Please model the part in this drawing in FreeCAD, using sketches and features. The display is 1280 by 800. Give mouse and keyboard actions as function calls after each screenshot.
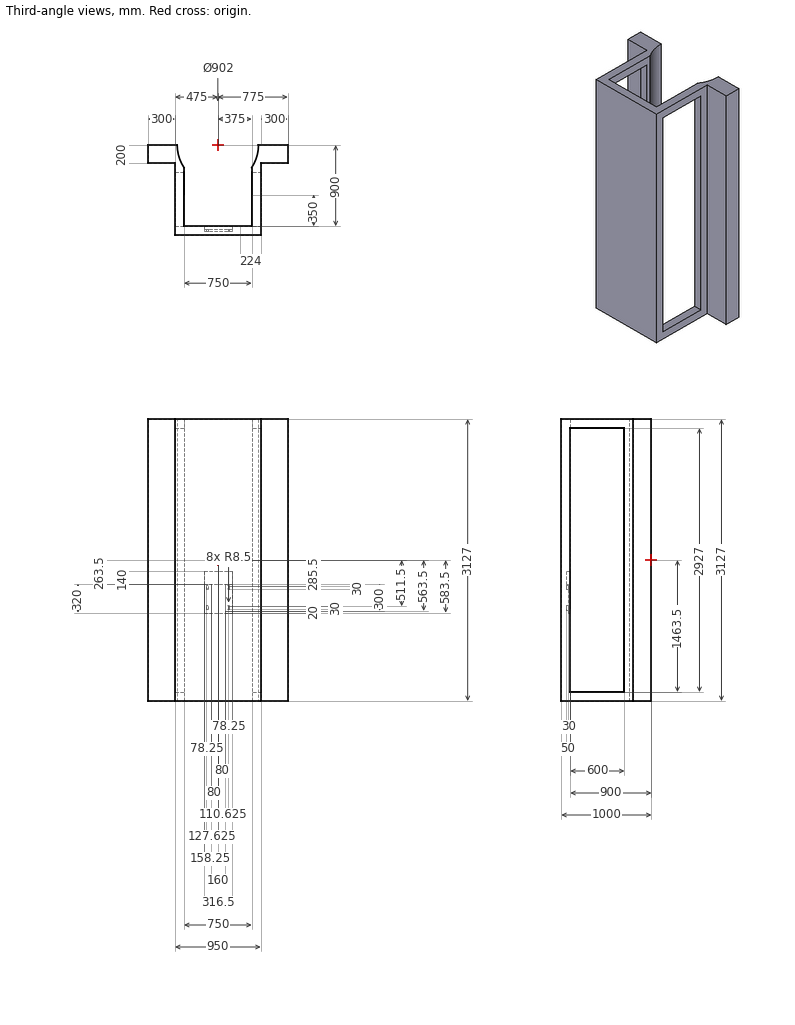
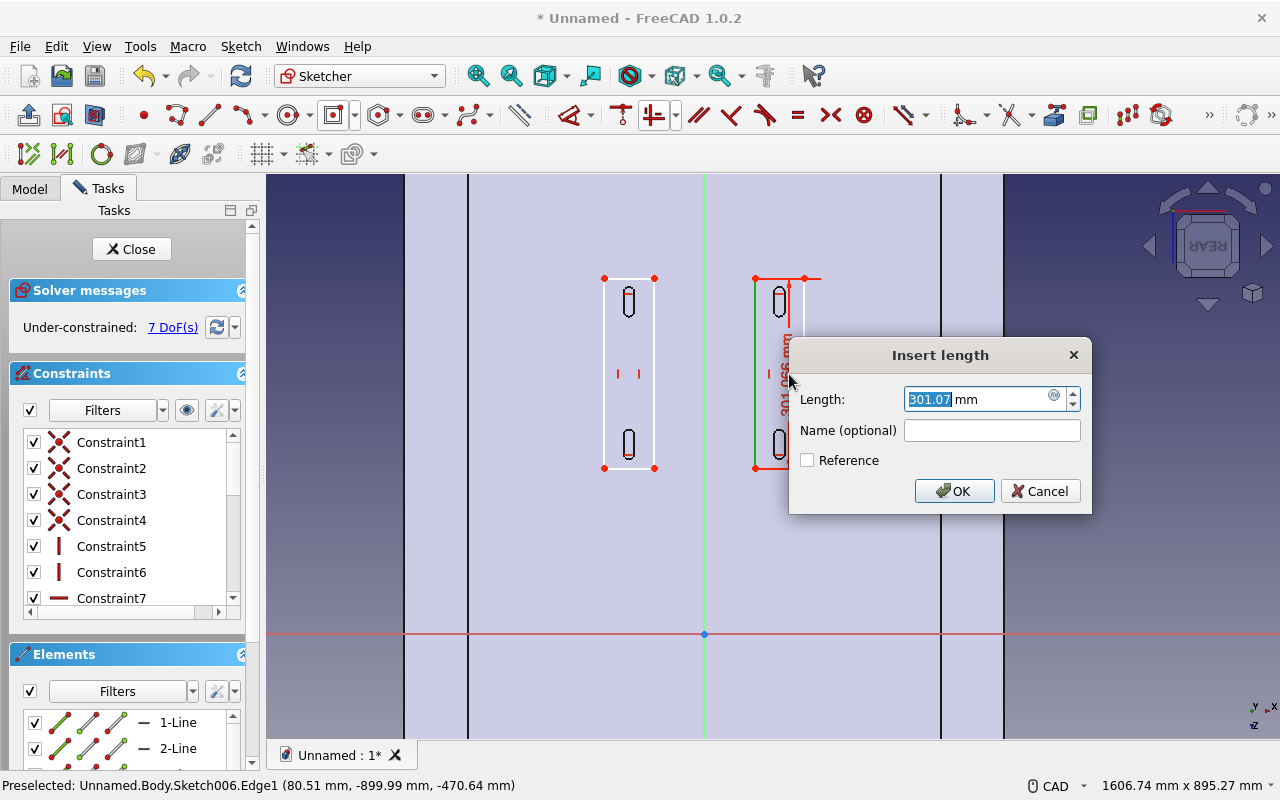
text(300)
key(Return)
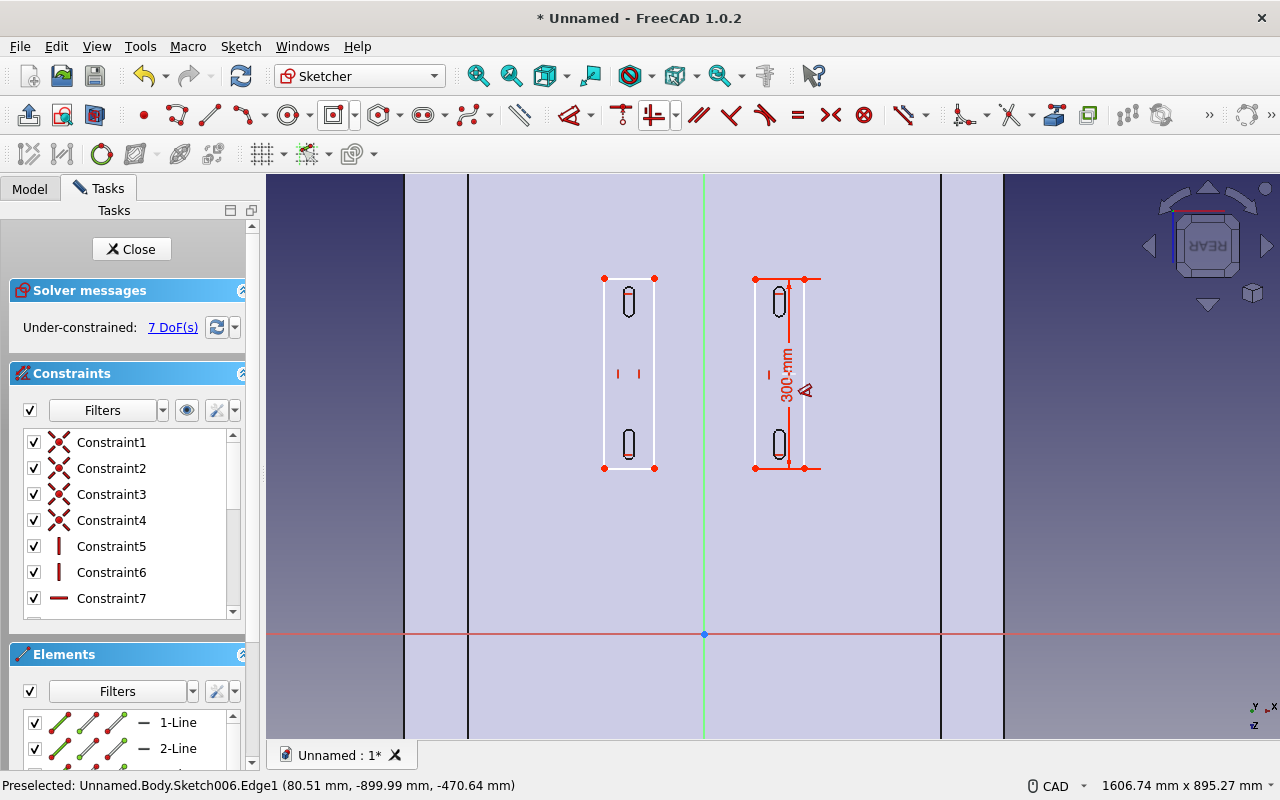
click(604, 336)
click(570, 374)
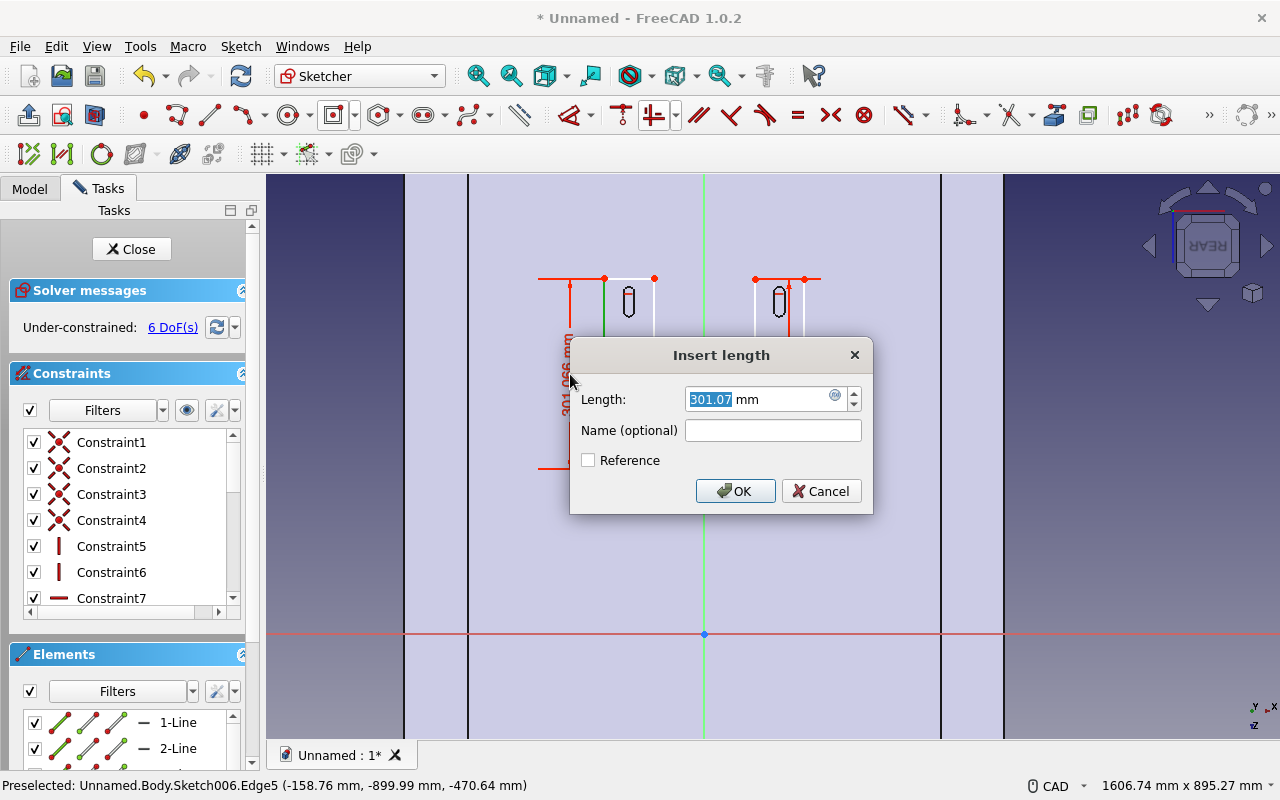
text(300)
key(Return)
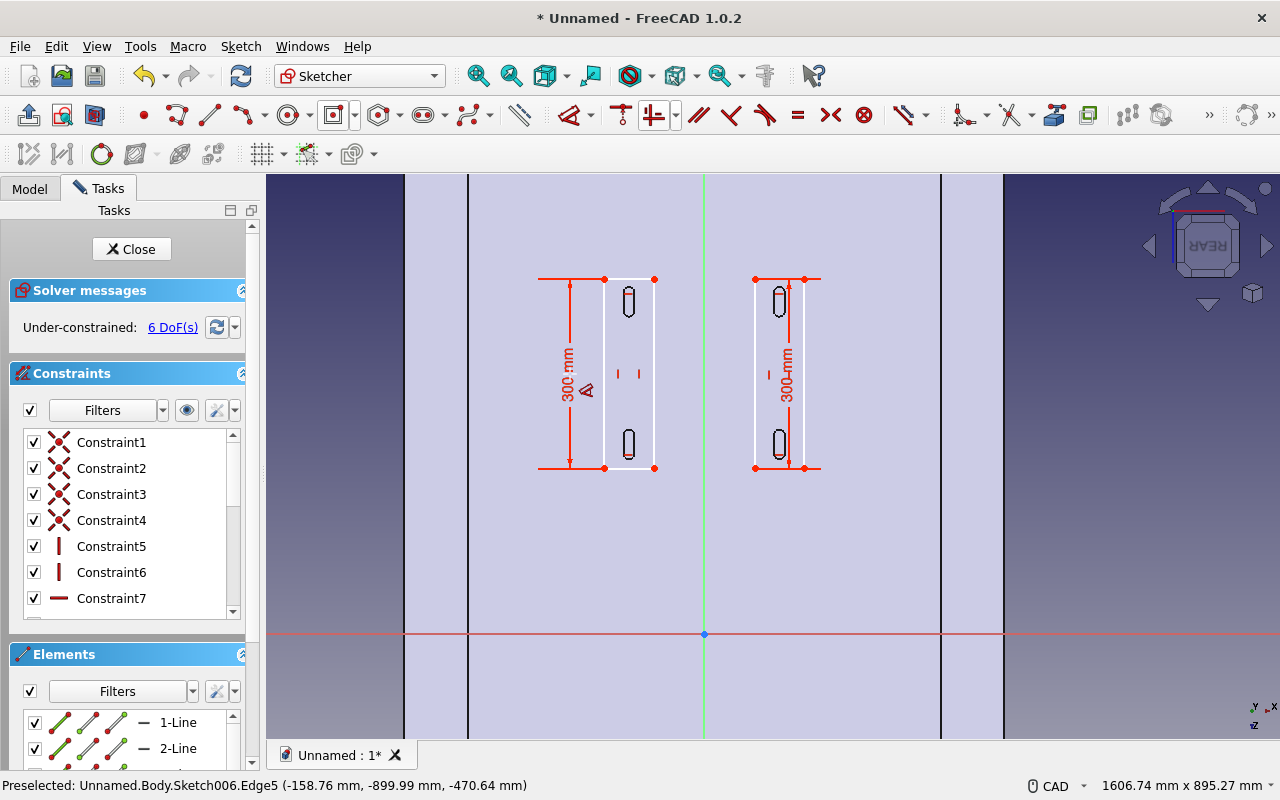
click(755, 279)
click(730, 668)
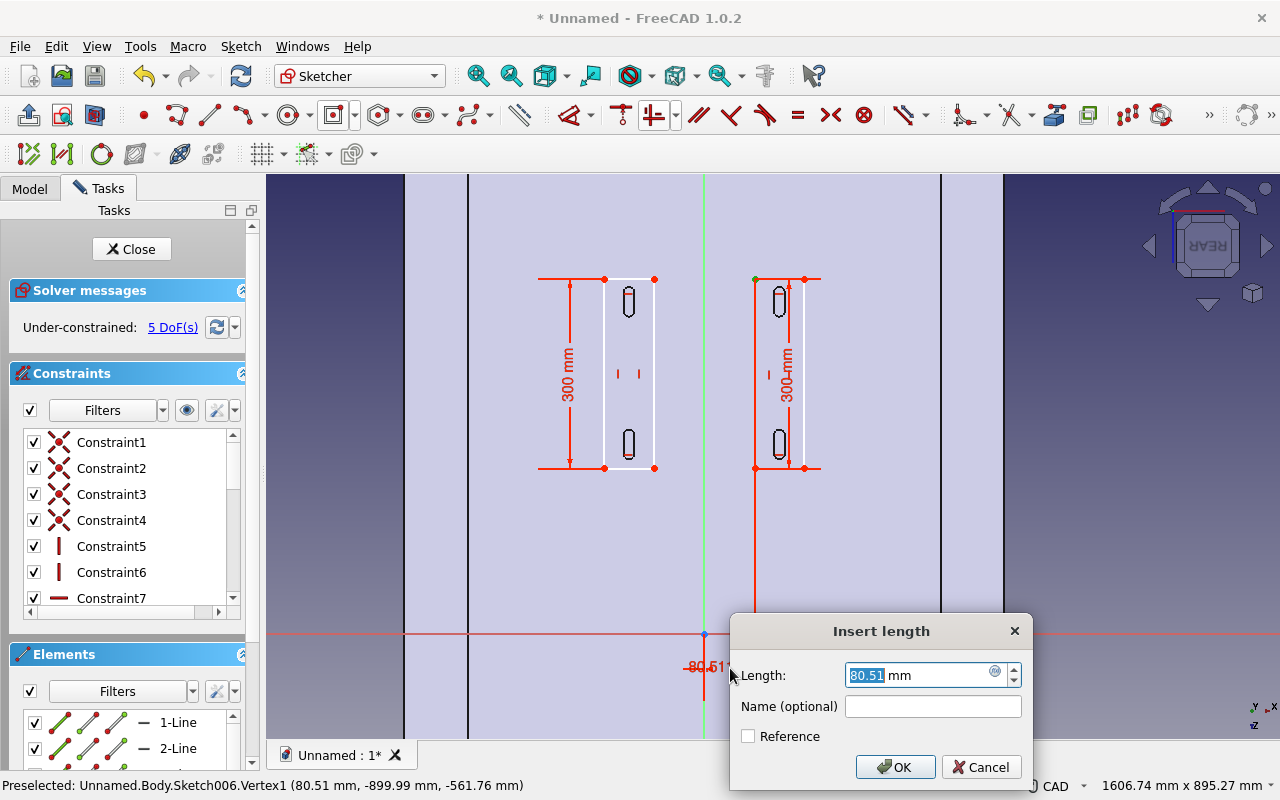
text(80)
key(Return)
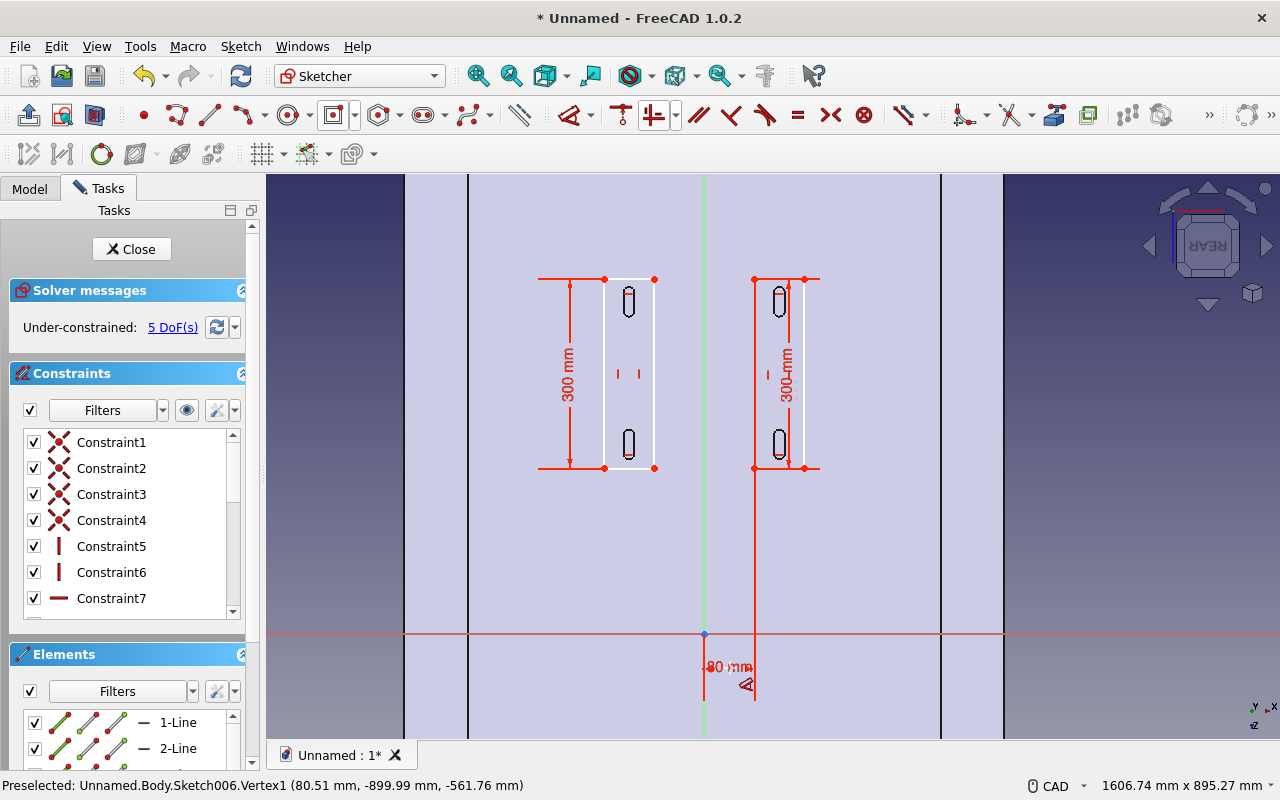
click(654, 469)
click(679, 435)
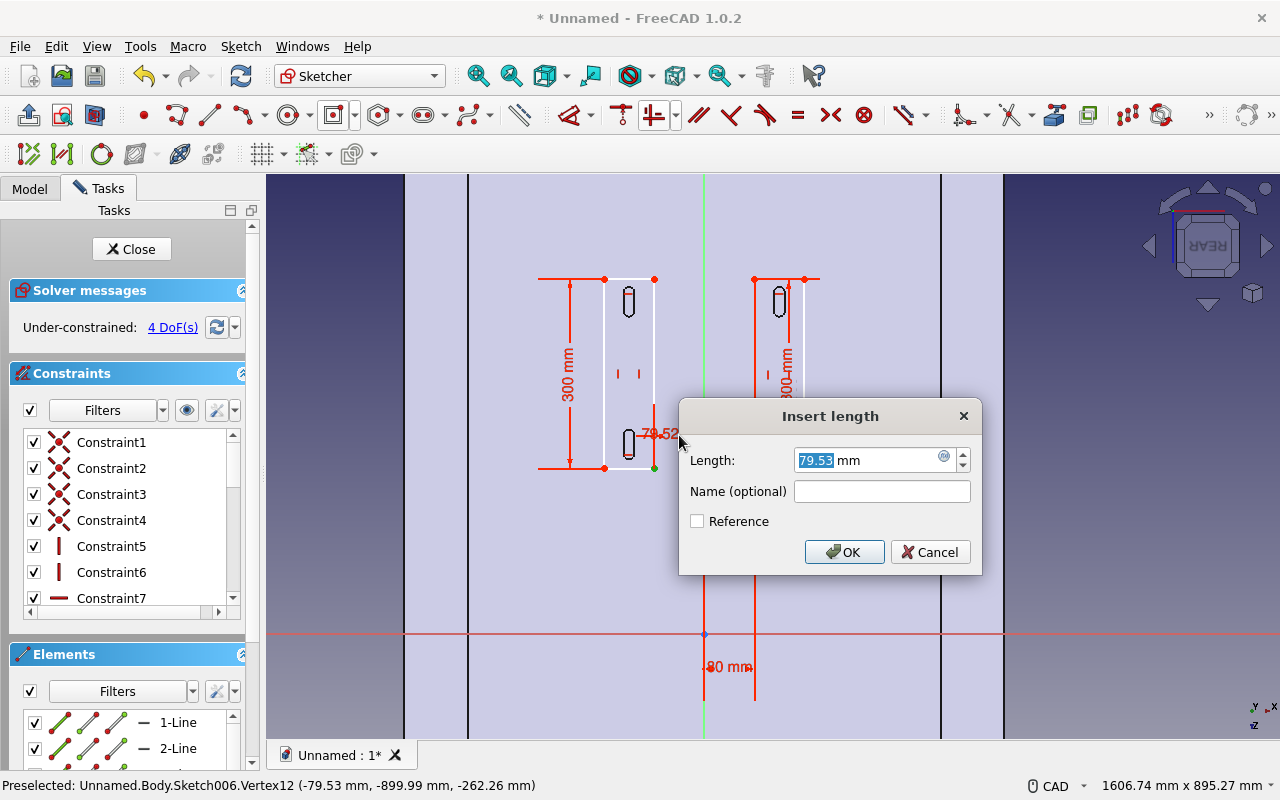
text(80)
key(Return)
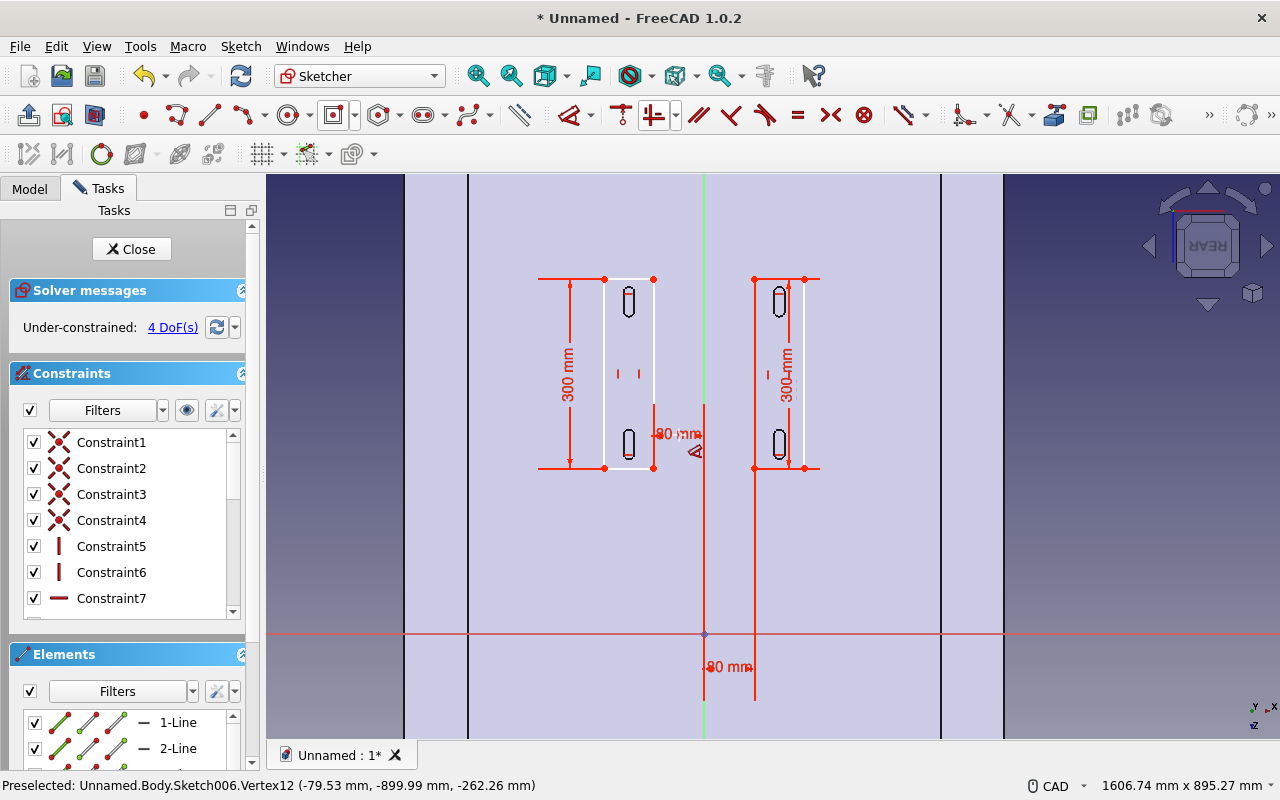
click(769, 469)
click(779, 503)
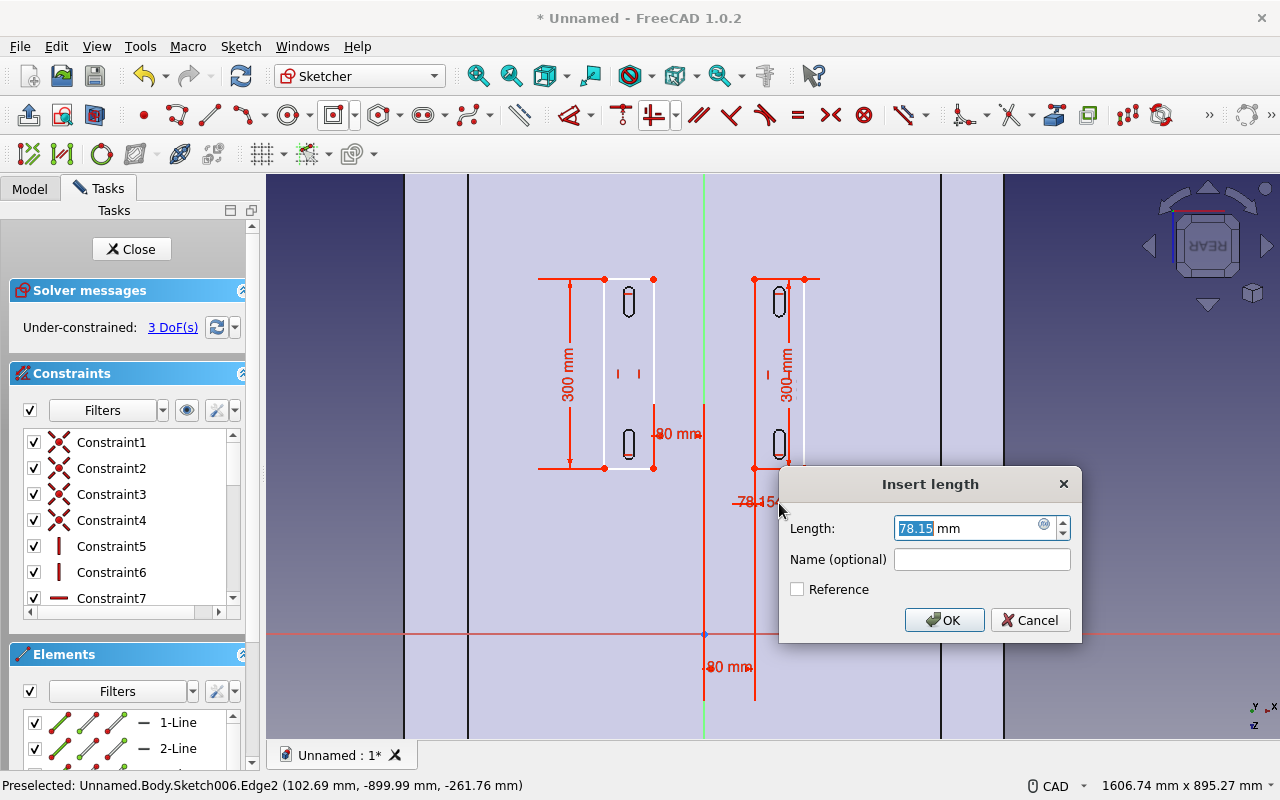
text(78.25)
key(Return)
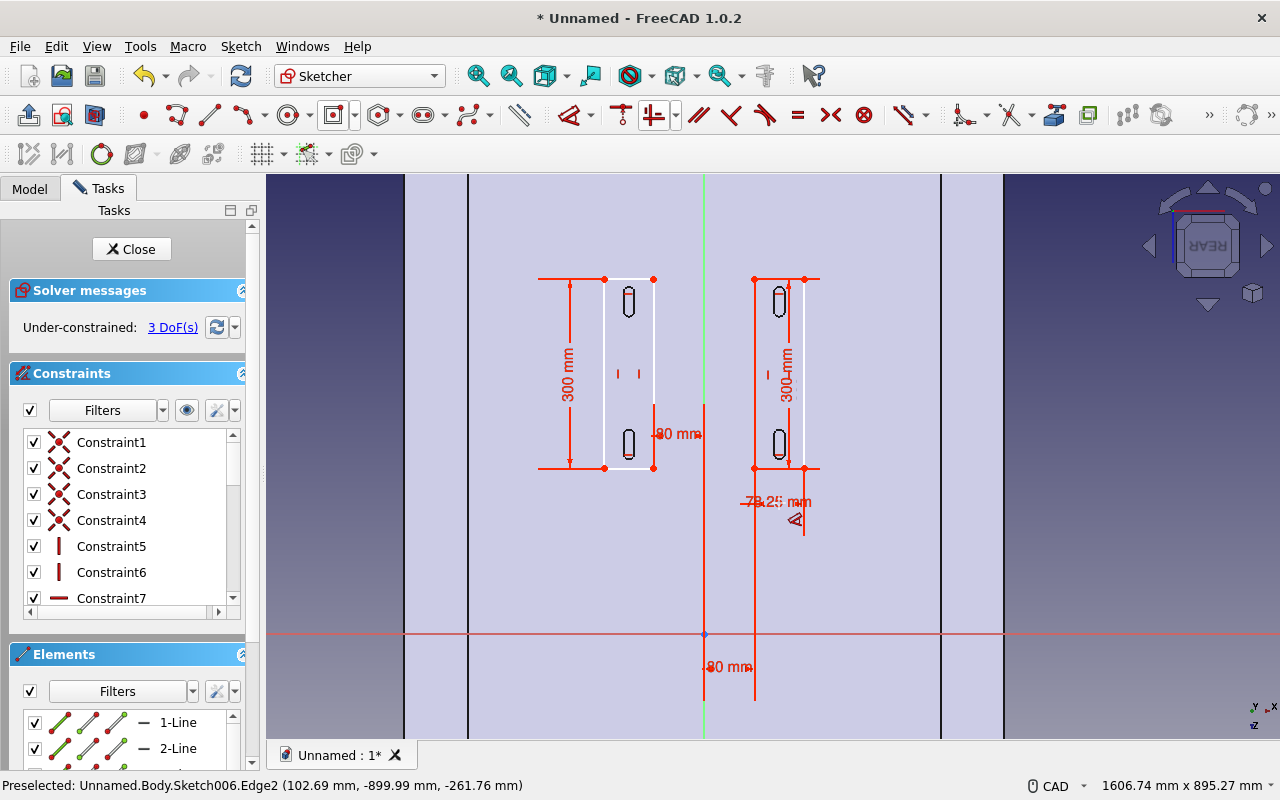
click(619, 469)
click(629, 503)